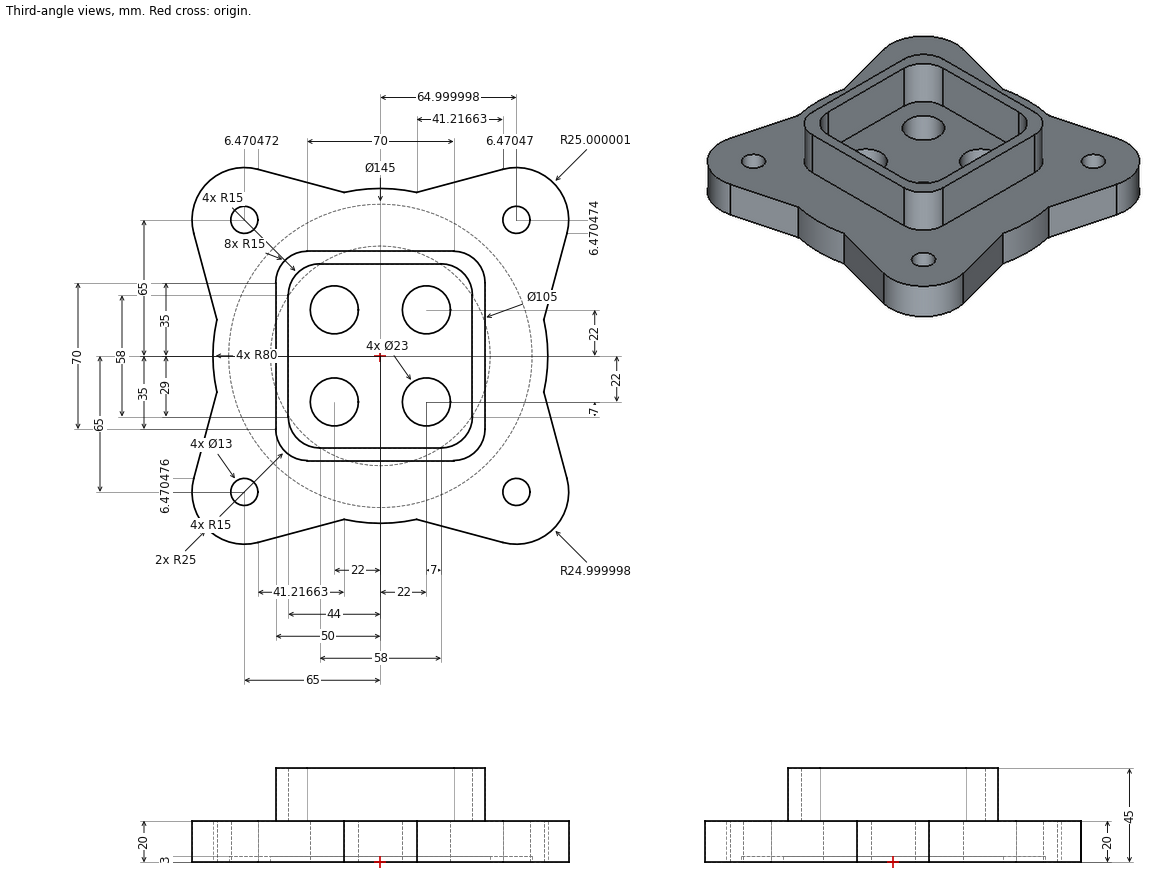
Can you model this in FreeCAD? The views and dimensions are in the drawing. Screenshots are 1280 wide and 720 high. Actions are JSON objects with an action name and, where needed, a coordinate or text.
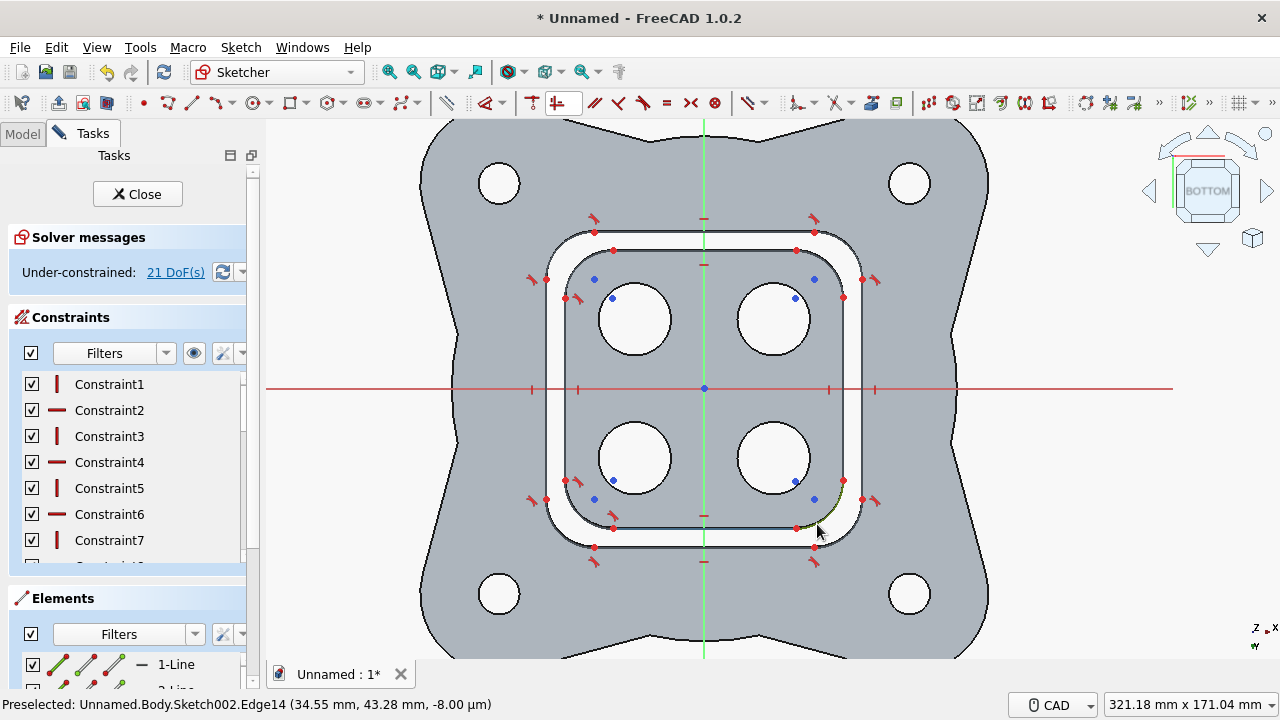
{"action": "left_click", "coordinate": [644, 104]}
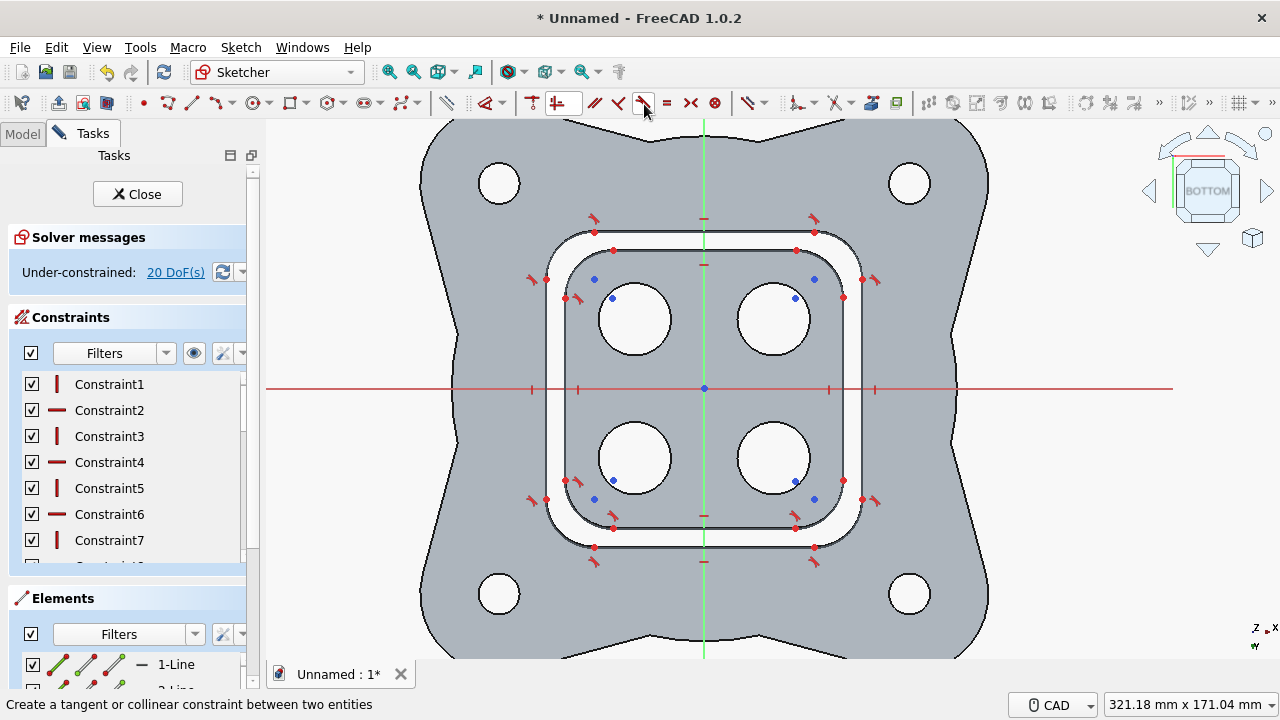
{"action": "left_click", "coordinate": [843, 426]}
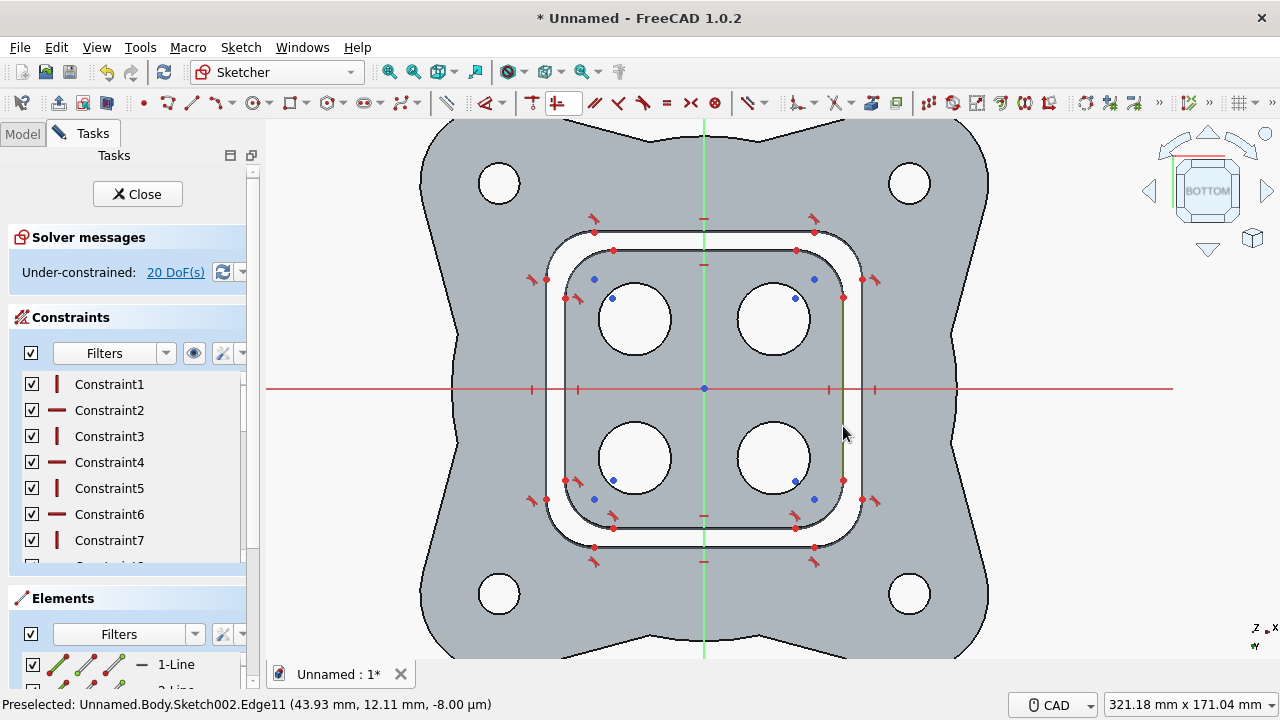
{"action": "left_click", "coordinate": [817, 524]}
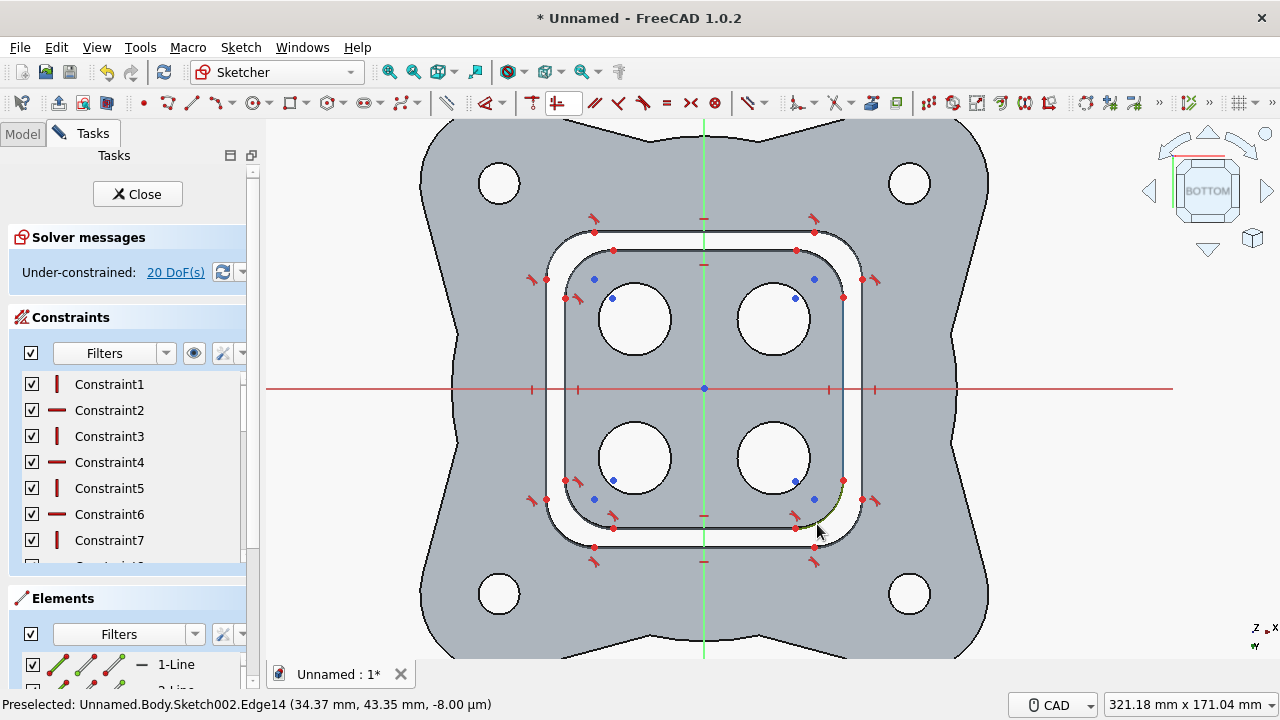
{"action": "left_click", "coordinate": [644, 104]}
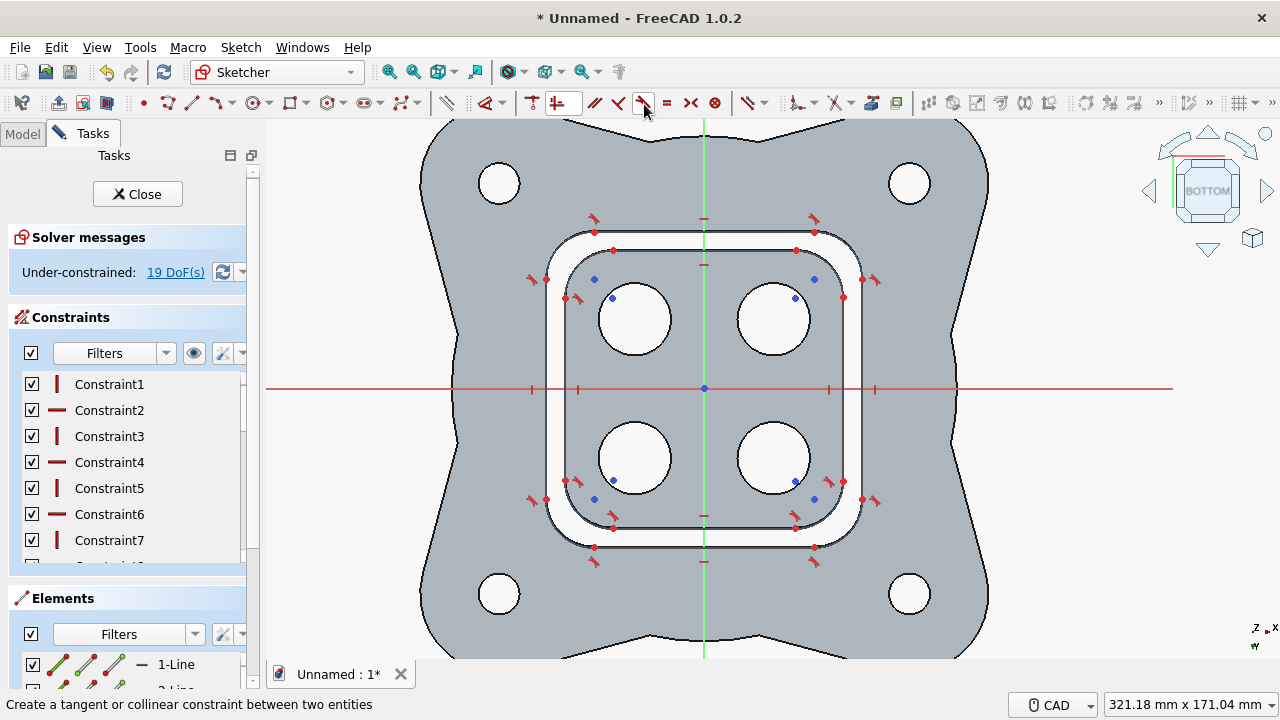
{"action": "left_click", "coordinate": [843, 426]}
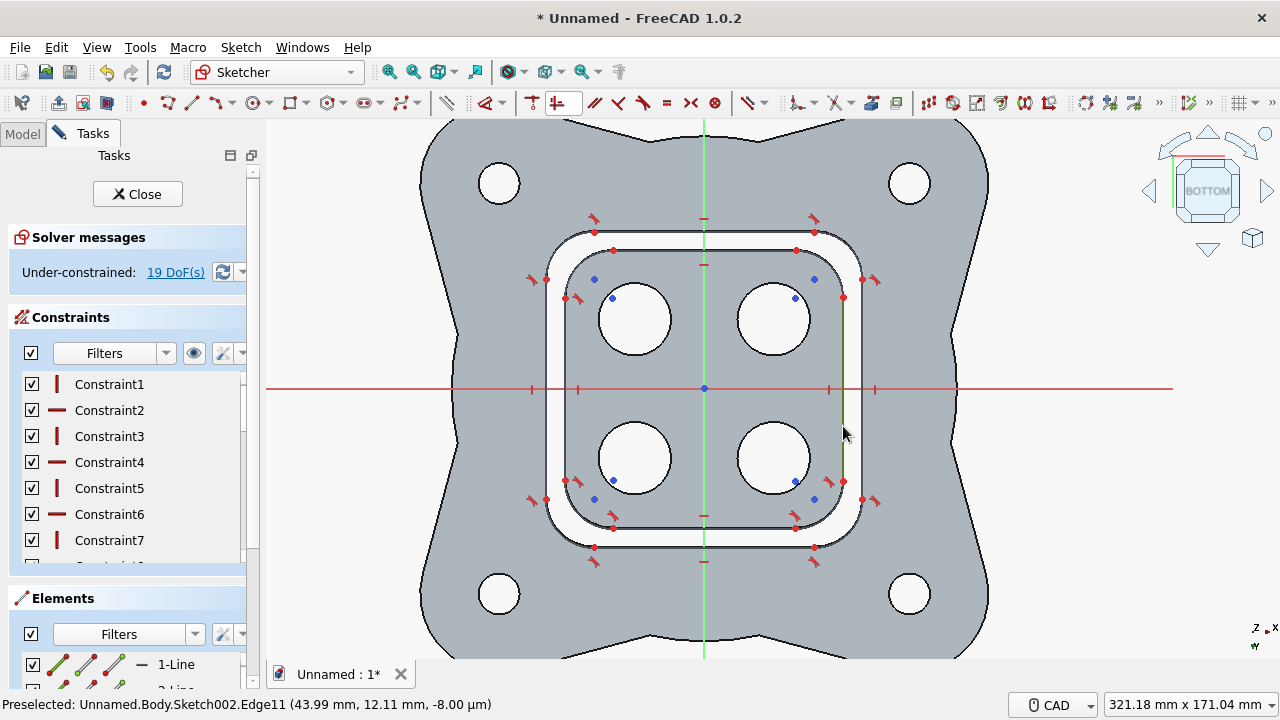
{"action": "left_click", "coordinate": [838, 277]}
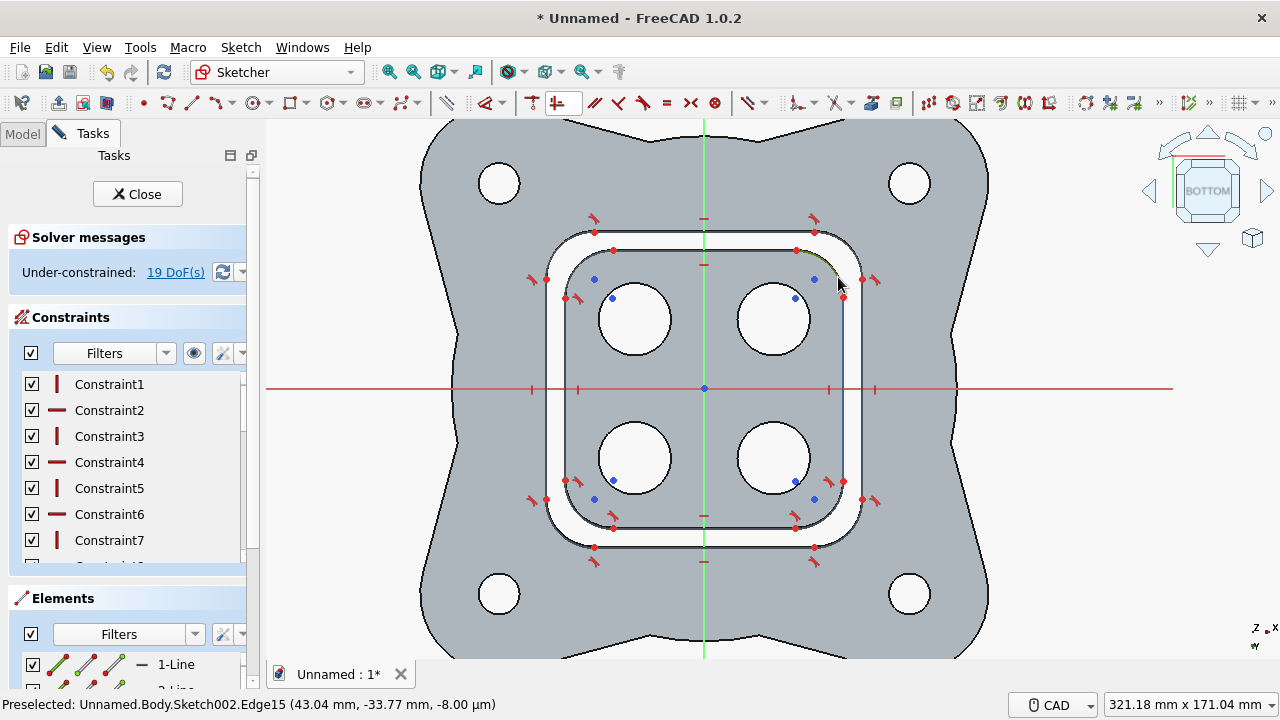
{"action": "left_click", "coordinate": [644, 104]}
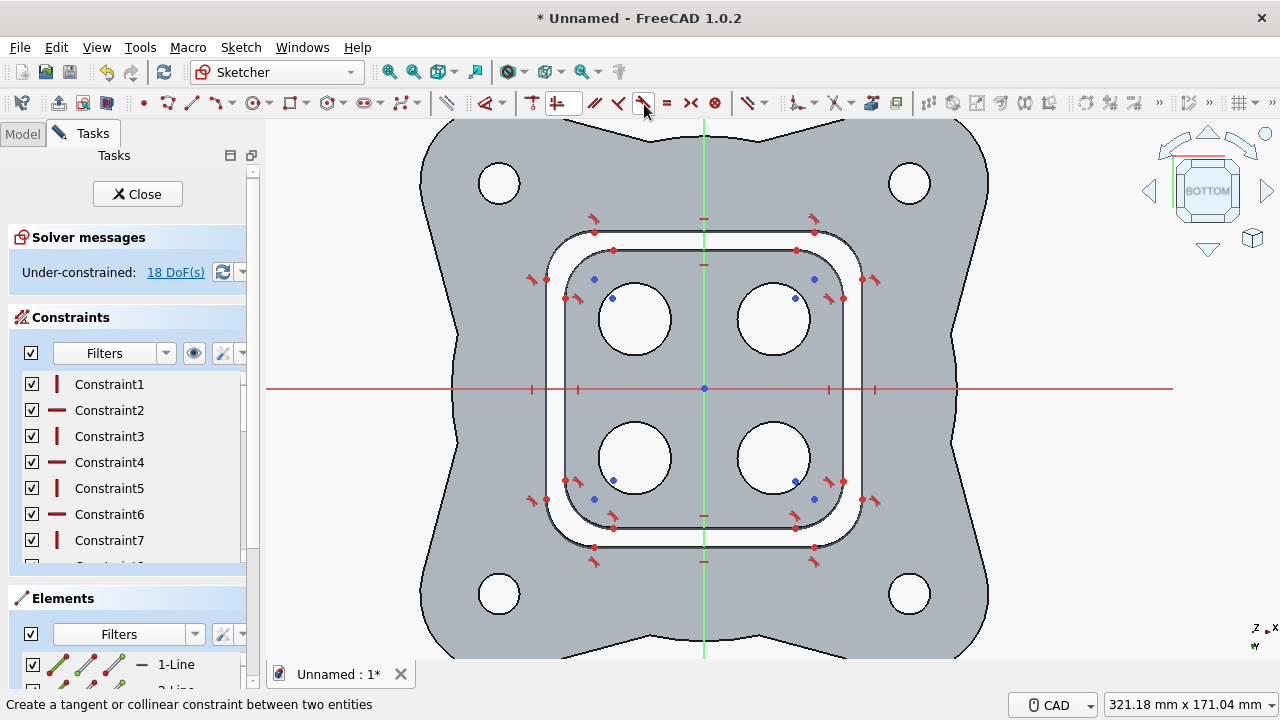
{"action": "left_click", "coordinate": [741, 251]}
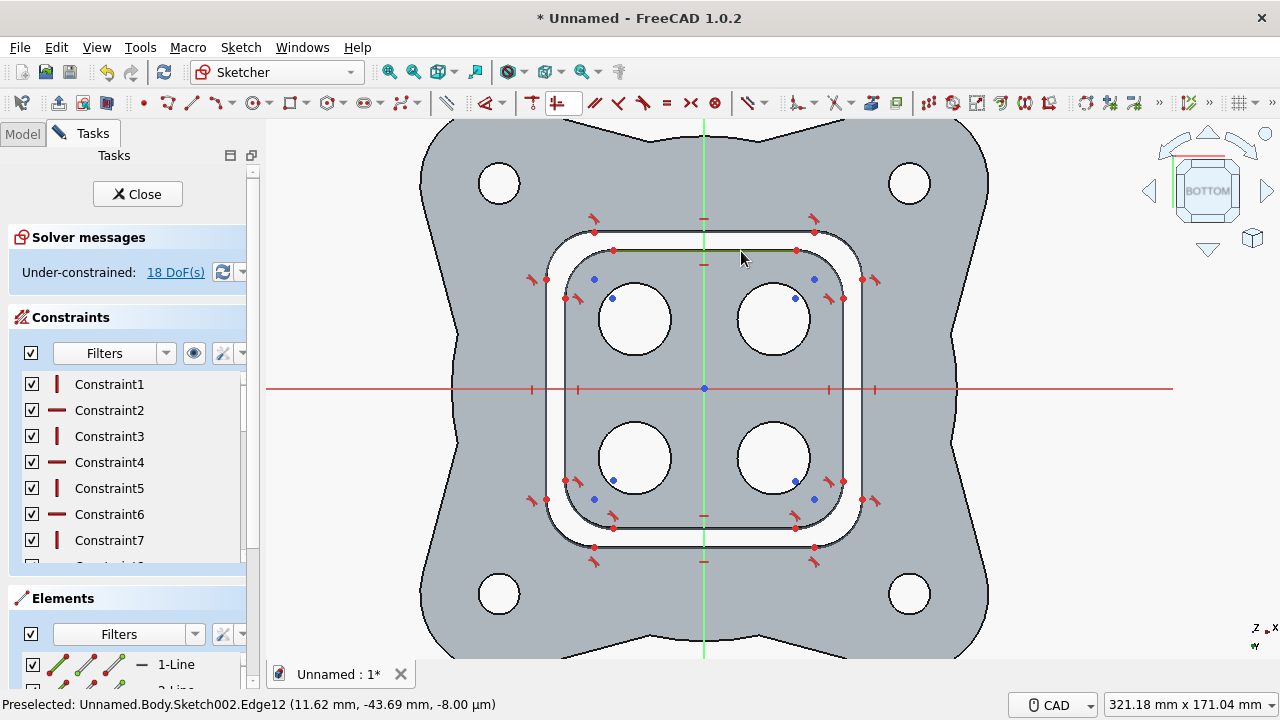
{"action": "left_click", "coordinate": [838, 277]}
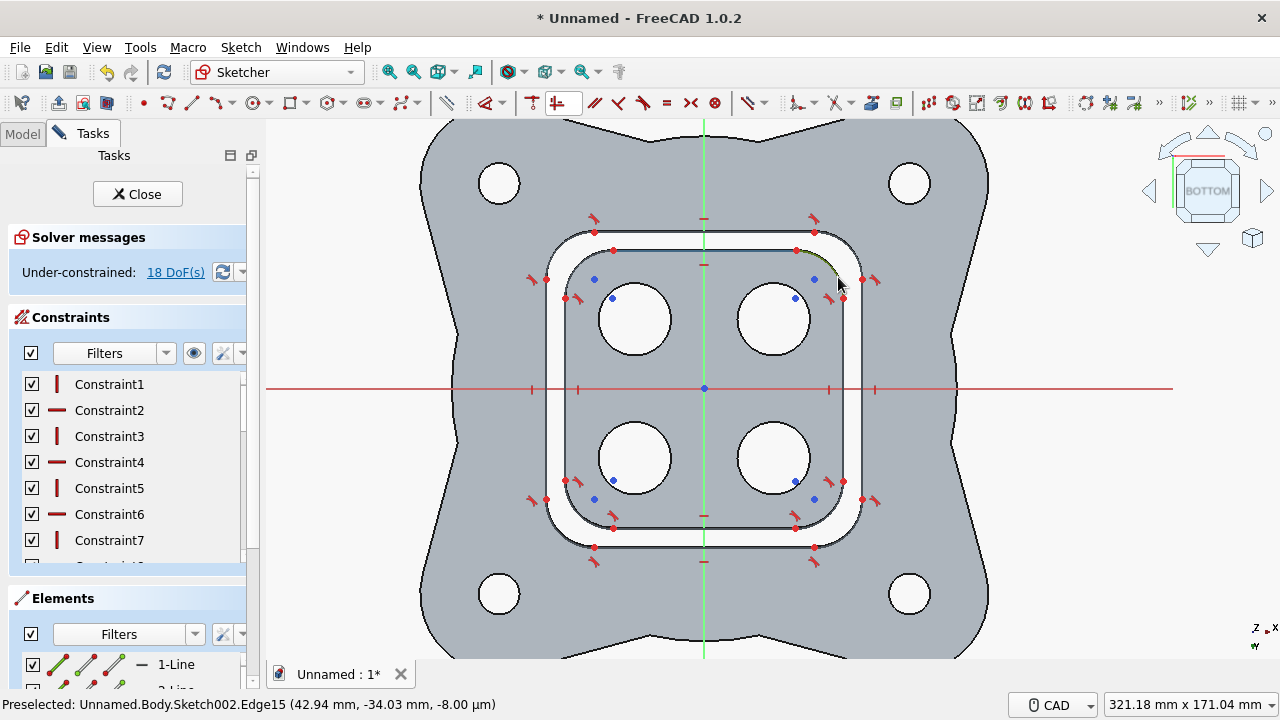
{"action": "left_click", "coordinate": [644, 104]}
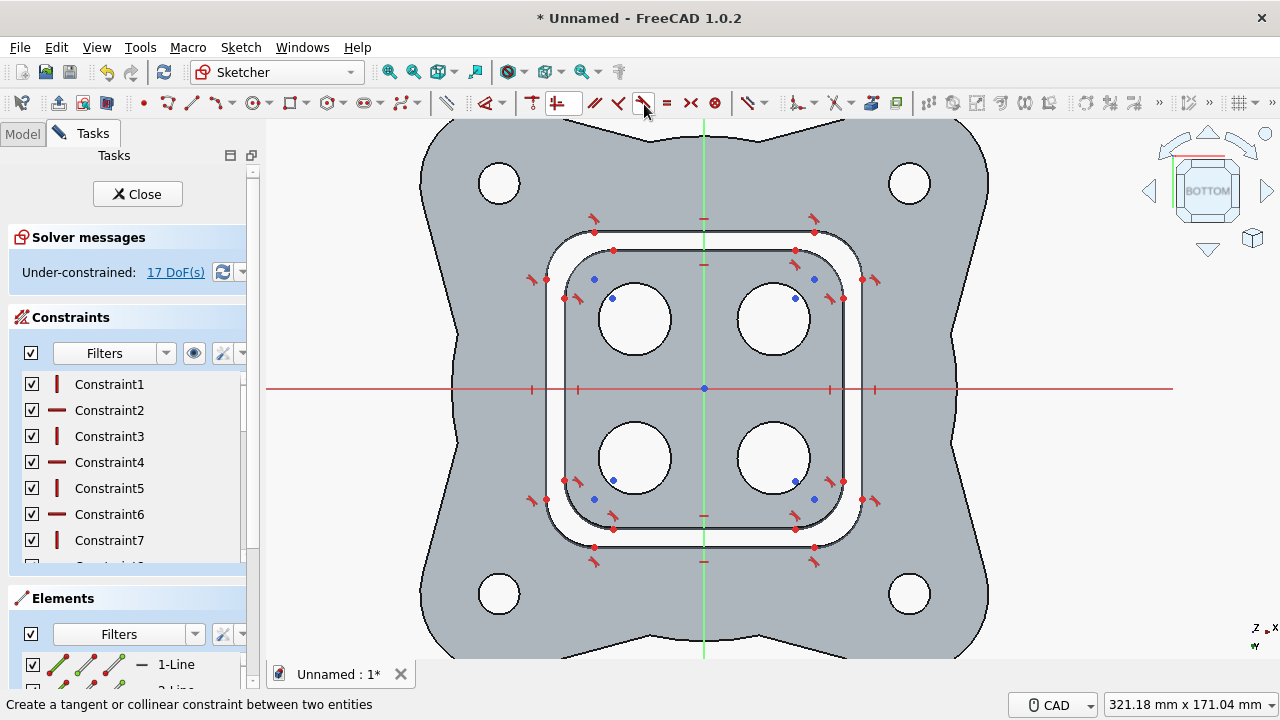
{"action": "left_click", "coordinate": [741, 251]}